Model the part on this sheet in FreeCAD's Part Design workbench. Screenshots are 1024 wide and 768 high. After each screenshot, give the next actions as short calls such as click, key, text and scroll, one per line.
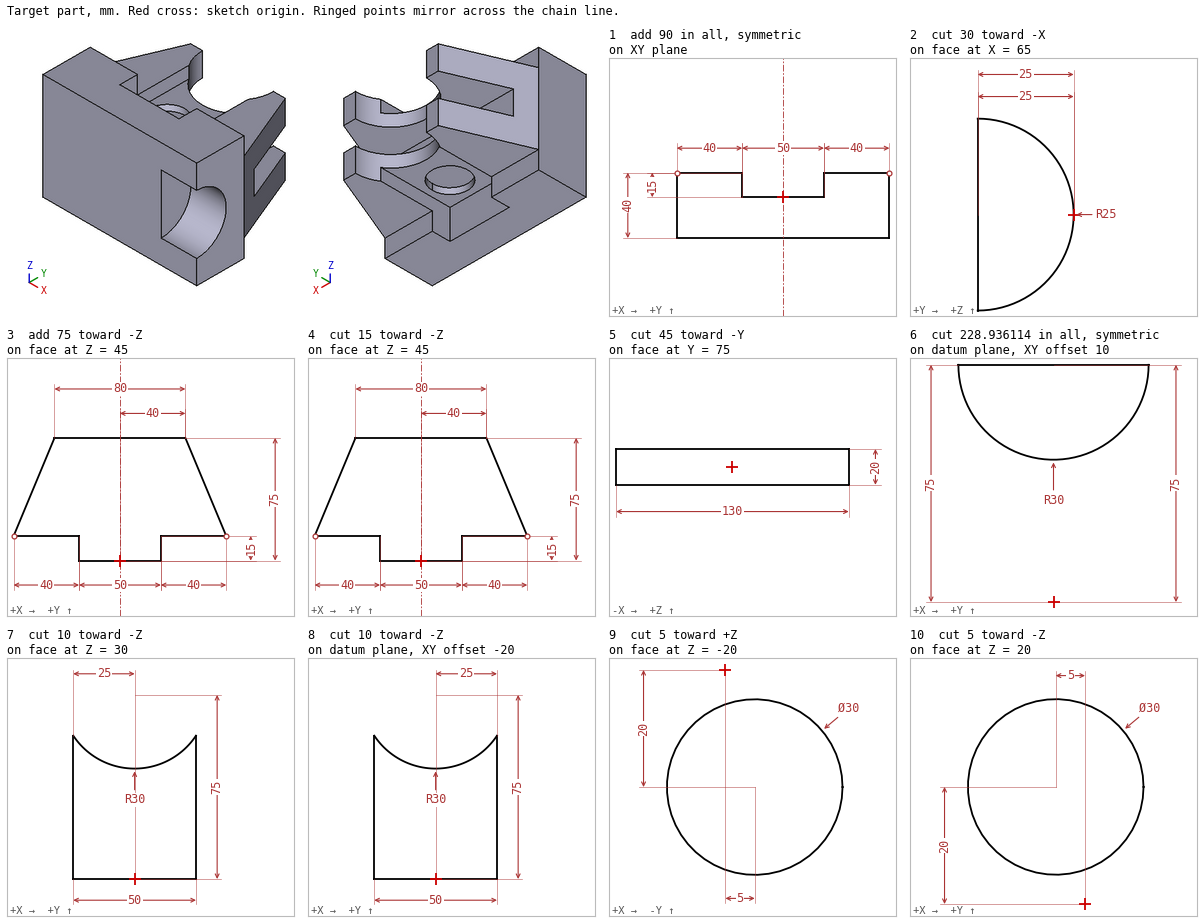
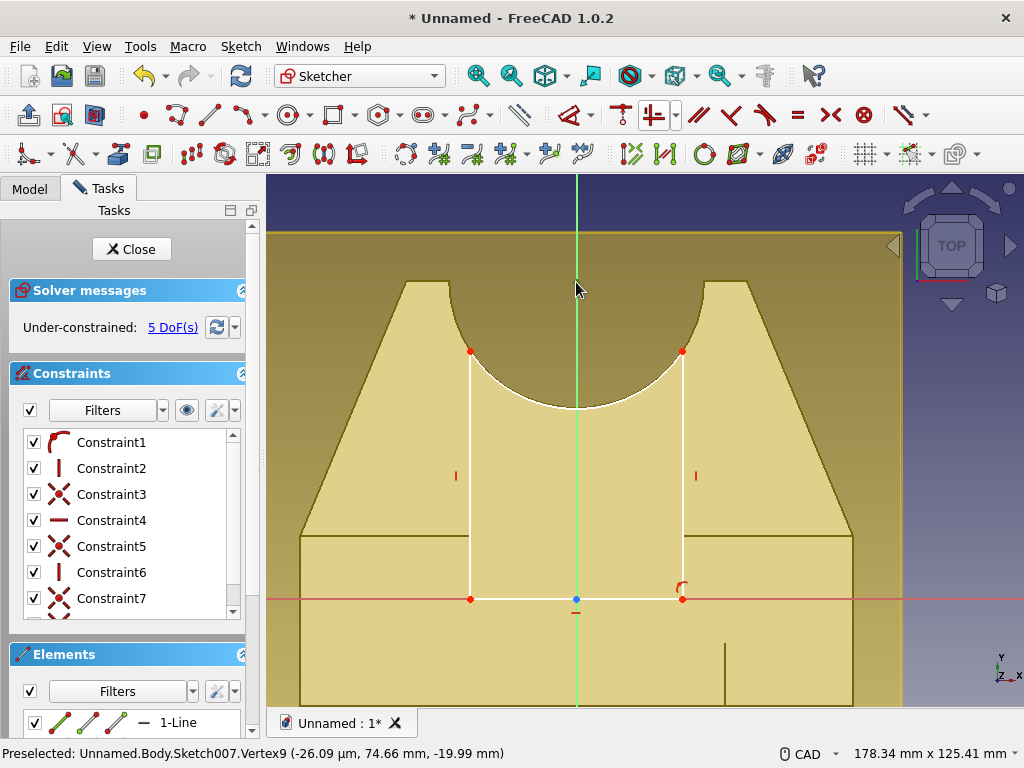
click(577, 645)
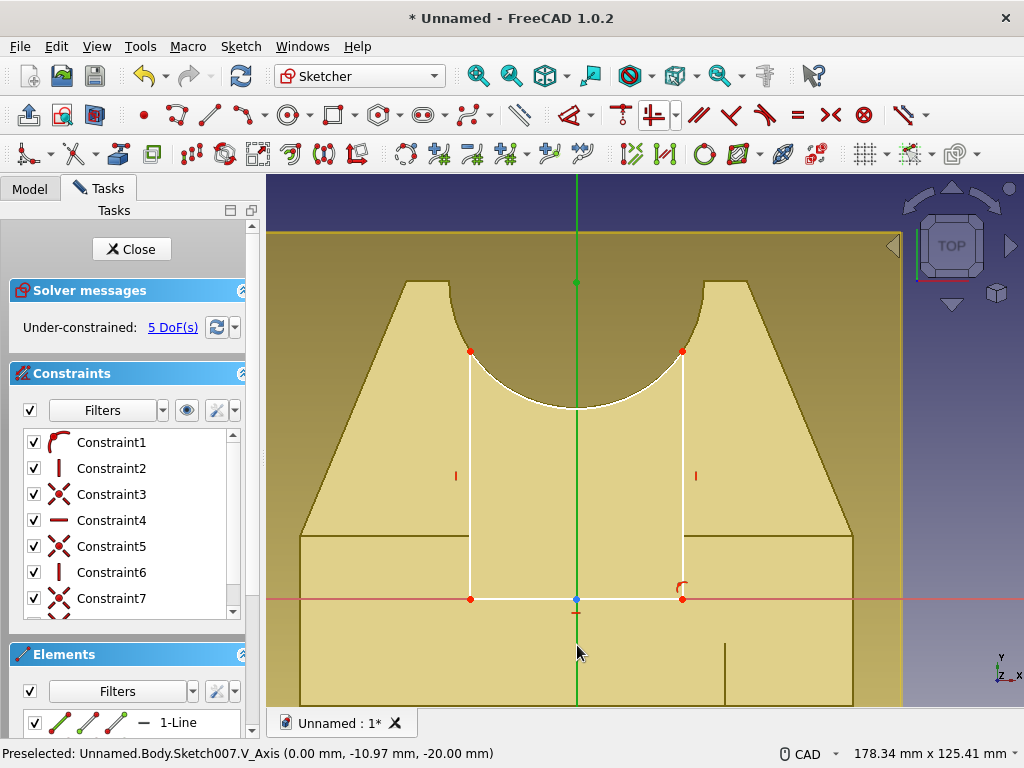
click(621, 116)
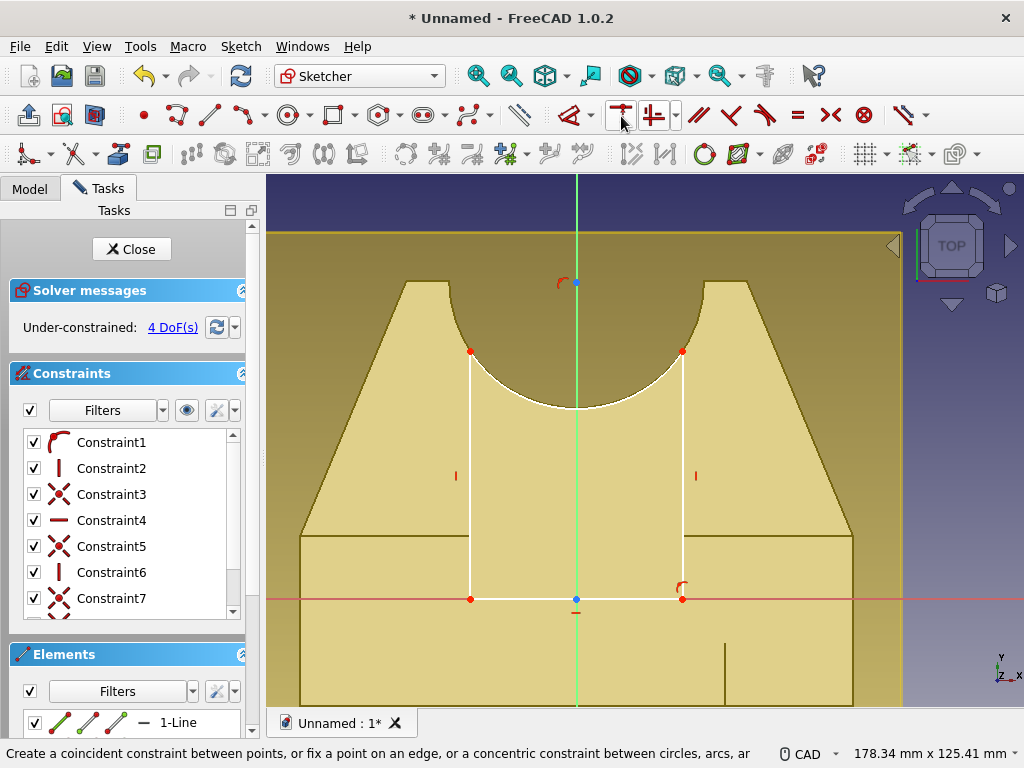
key(d)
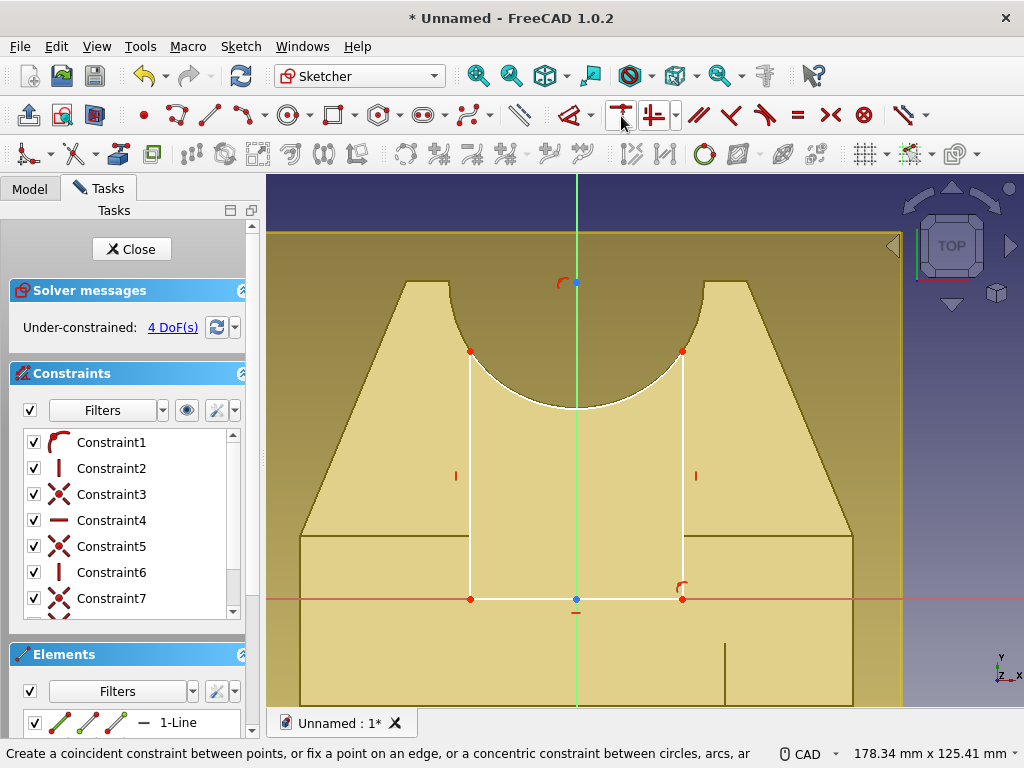
click(527, 399)
click(515, 428)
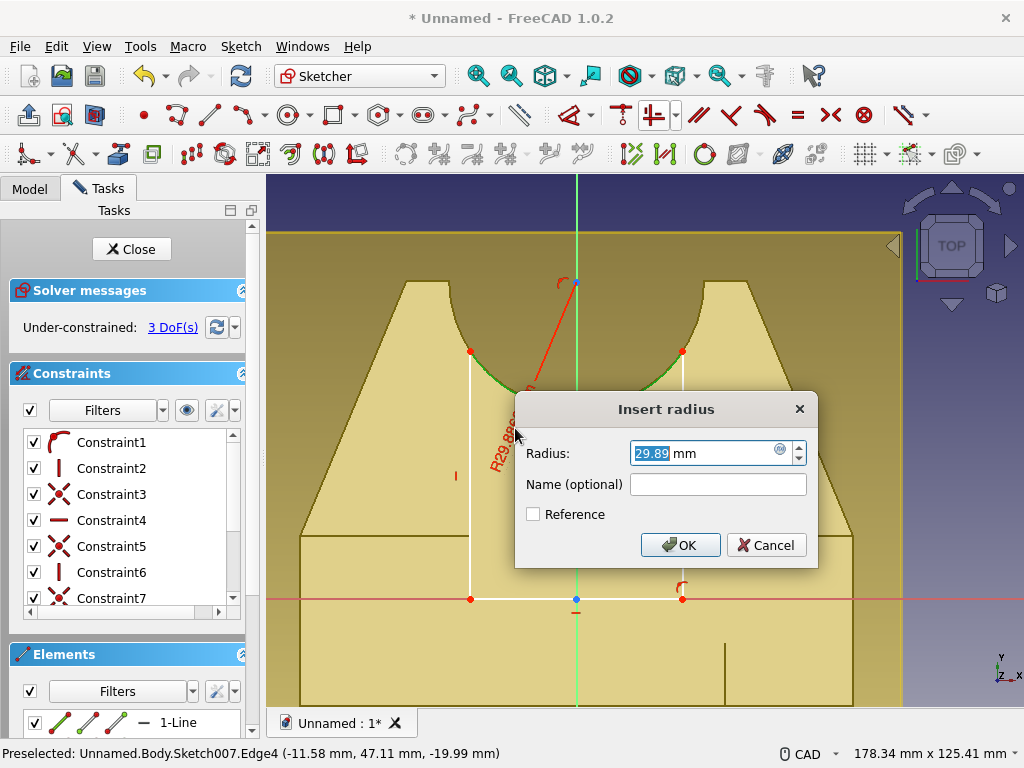
text(30)
key(Return)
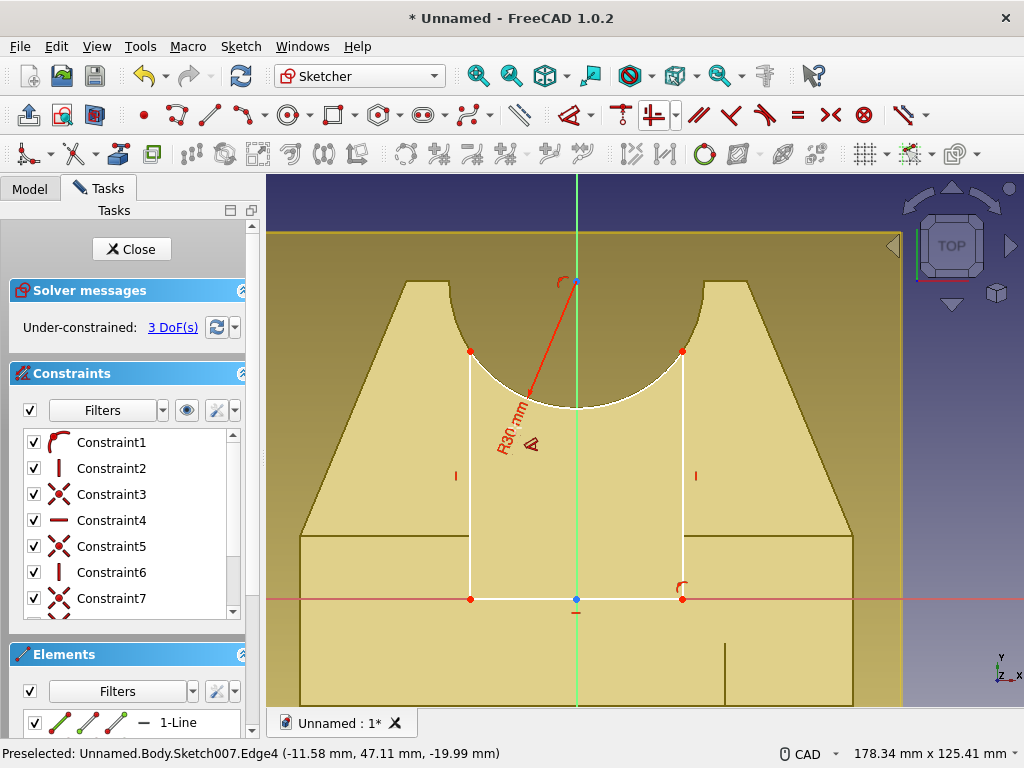
click(619, 599)
click(528, 633)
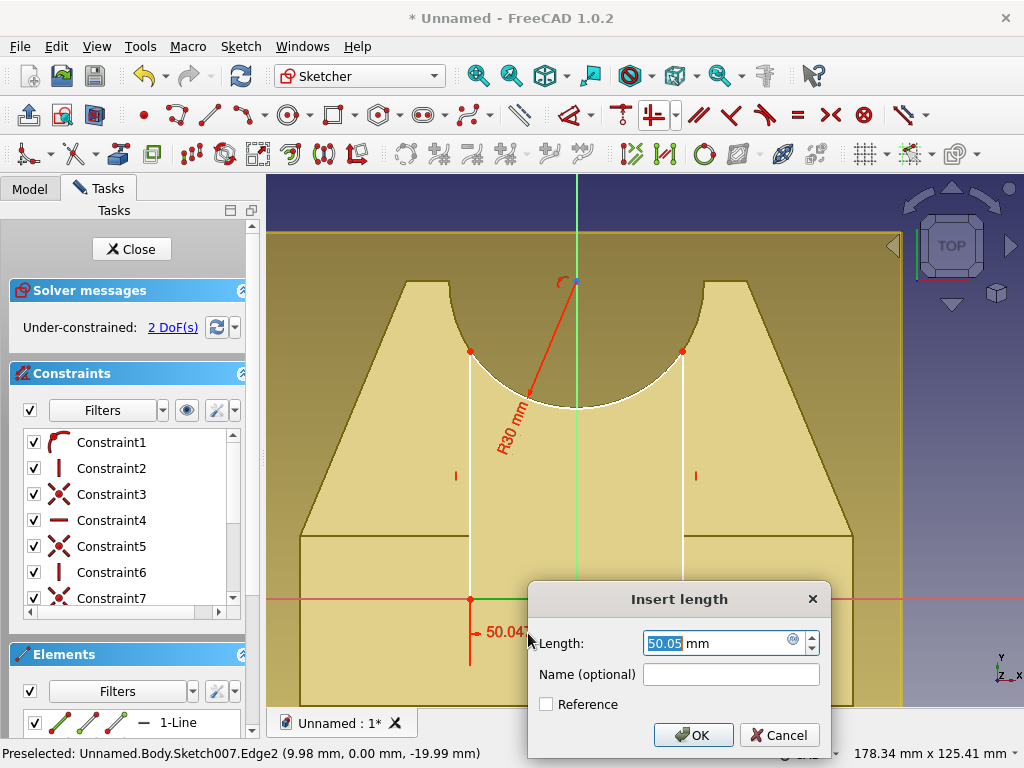
text(50)
key(Return)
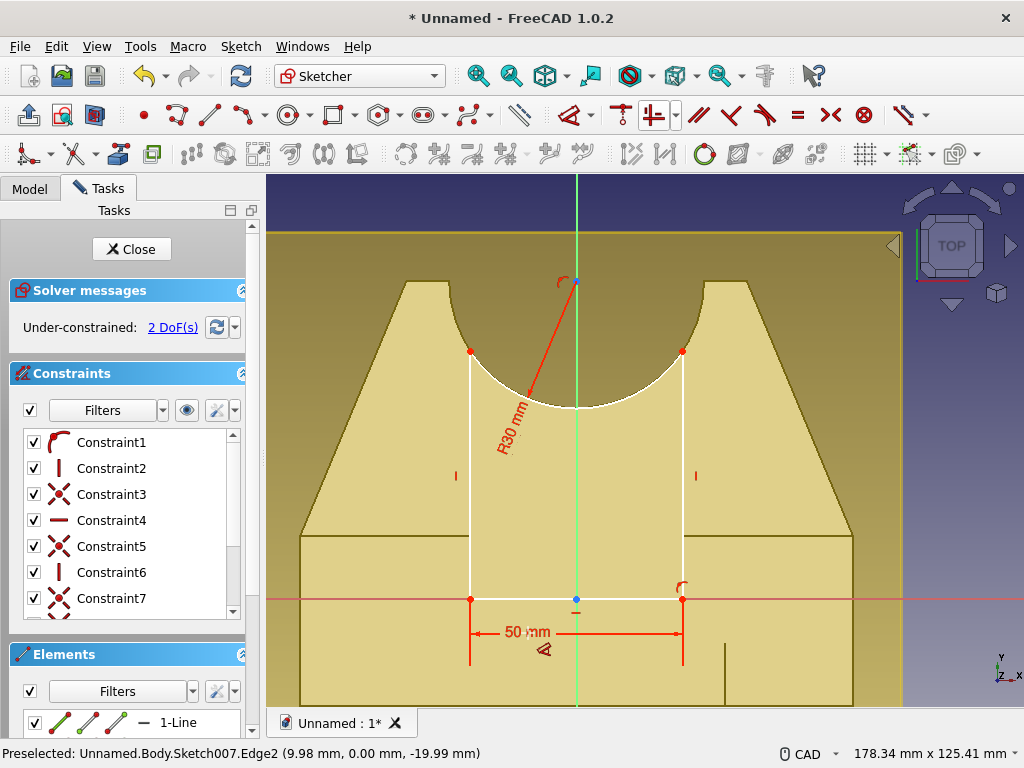
click(683, 351)
click(630, 633)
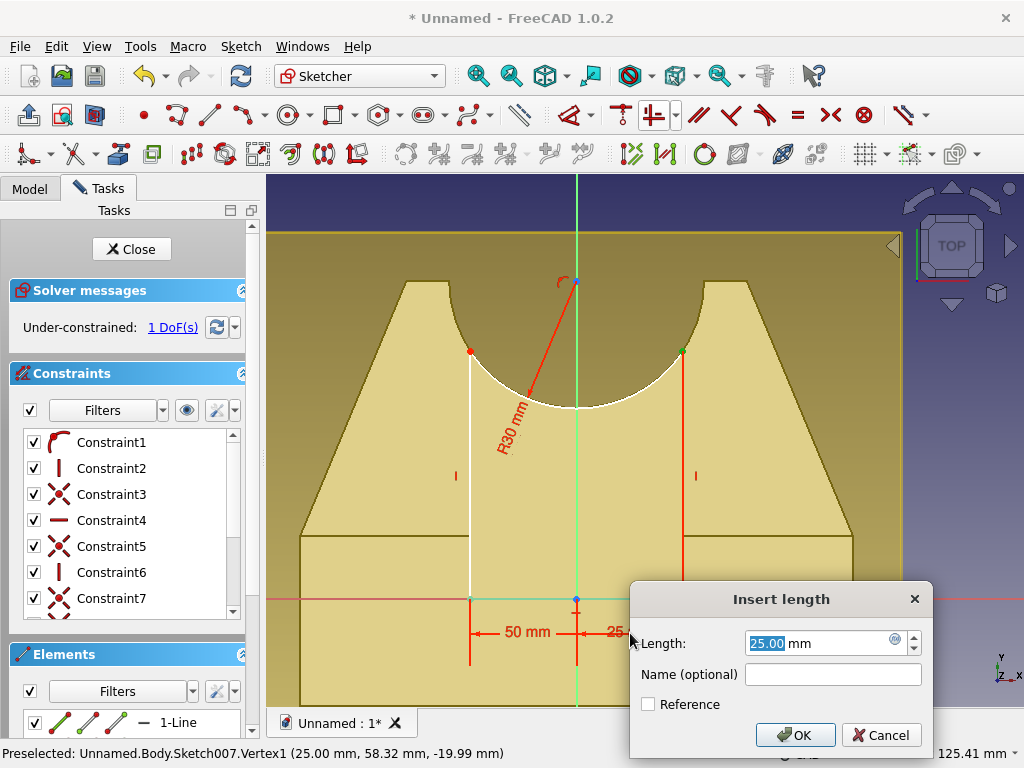
text(25)
key(Return)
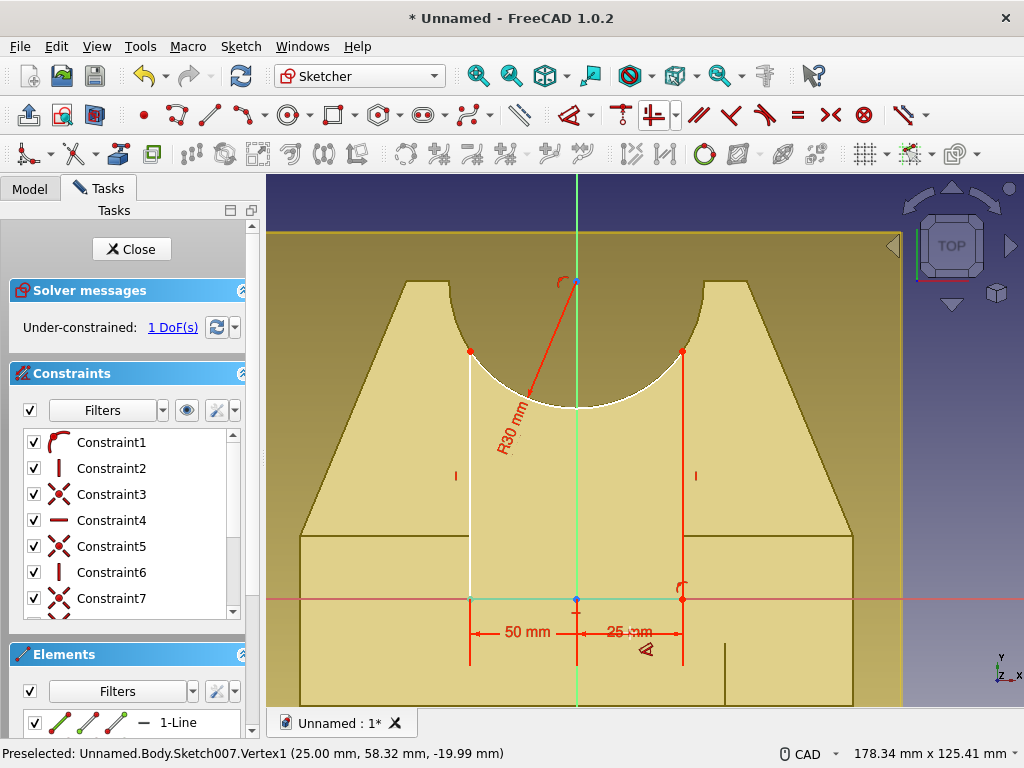
click(577, 281)
click(611, 440)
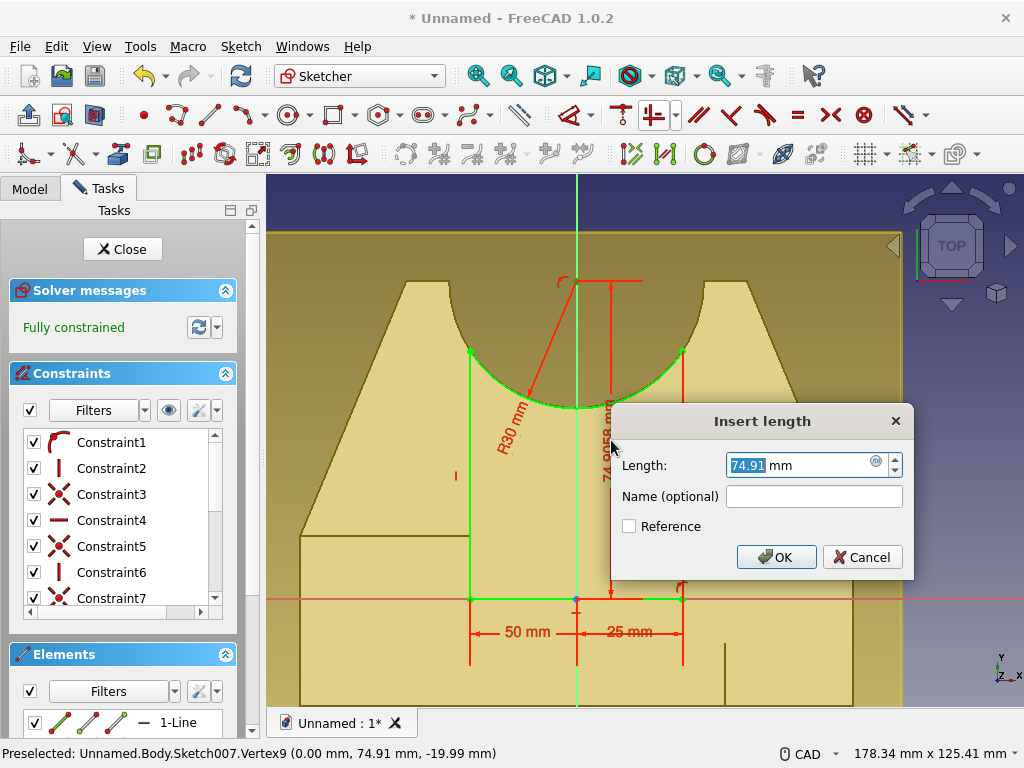
text(75)
key(Return)
key(Escape)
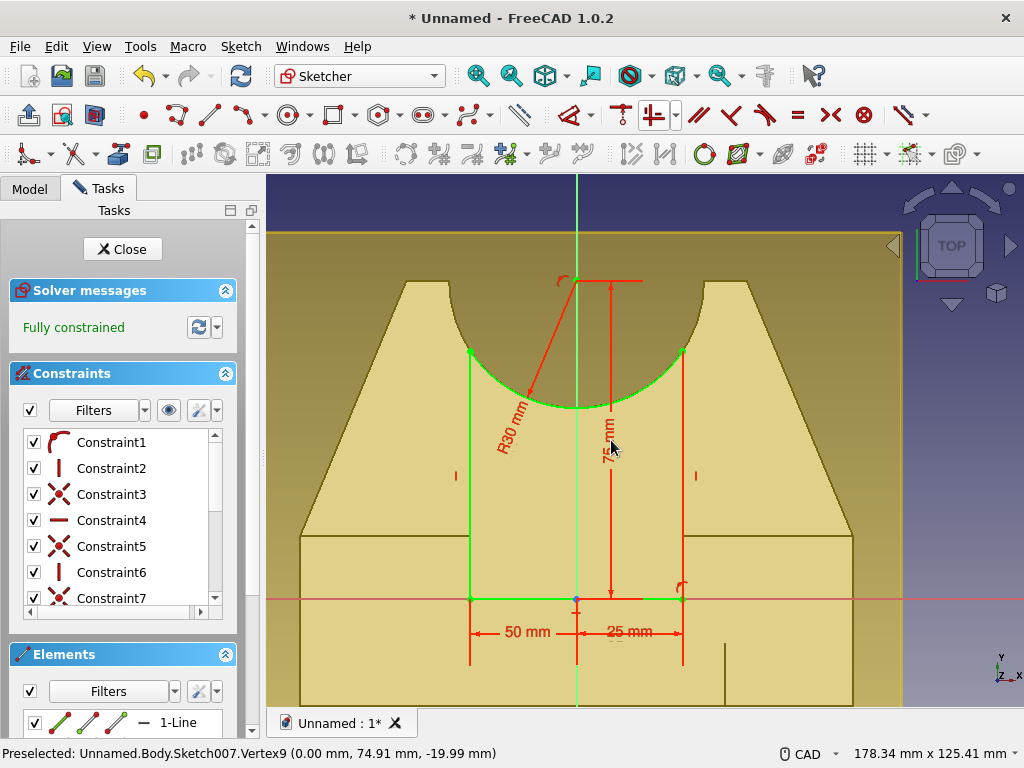
click(123, 249)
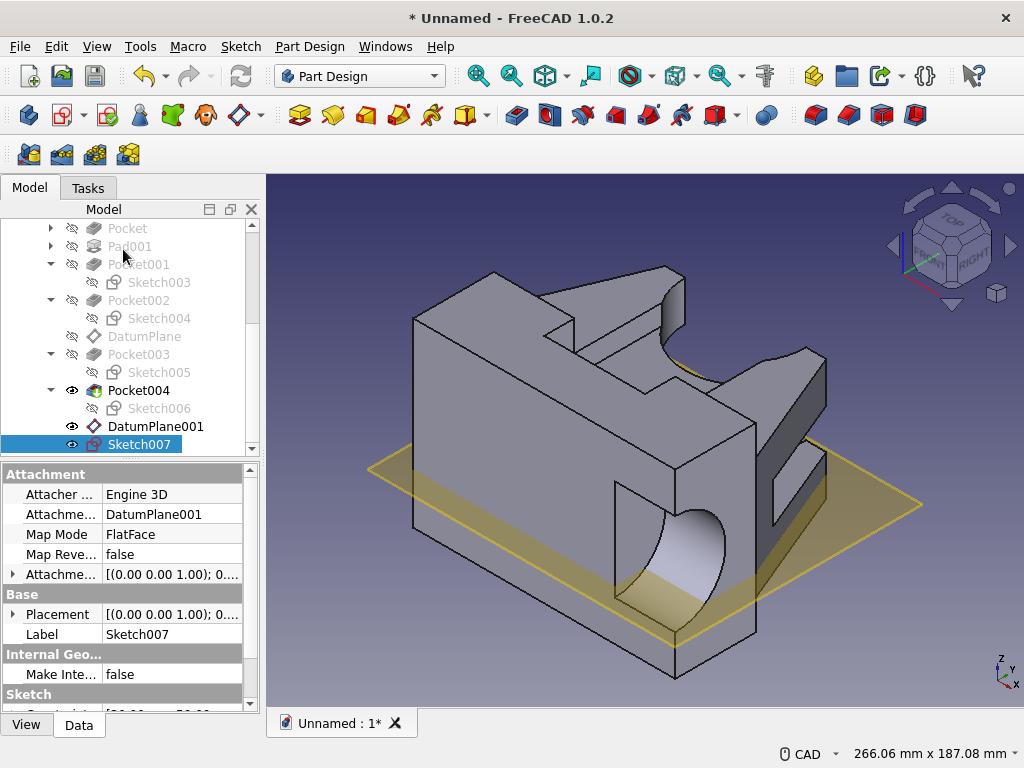
click(517, 116)